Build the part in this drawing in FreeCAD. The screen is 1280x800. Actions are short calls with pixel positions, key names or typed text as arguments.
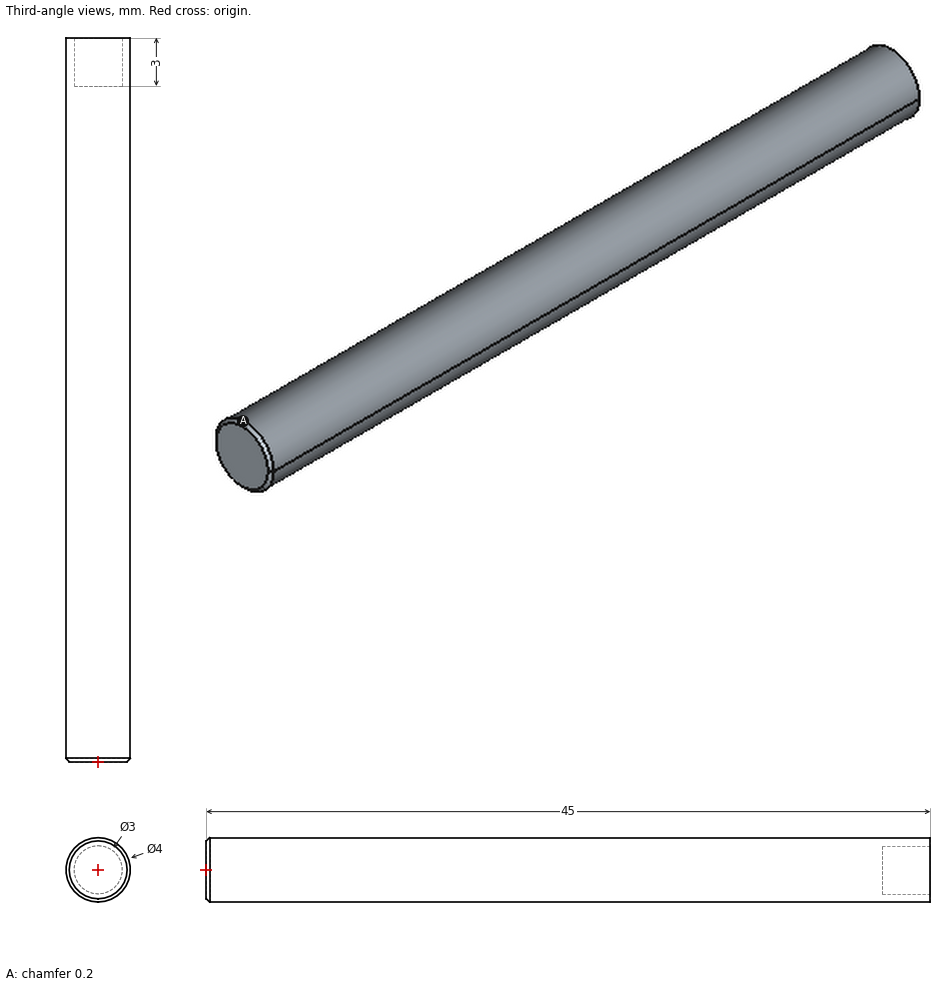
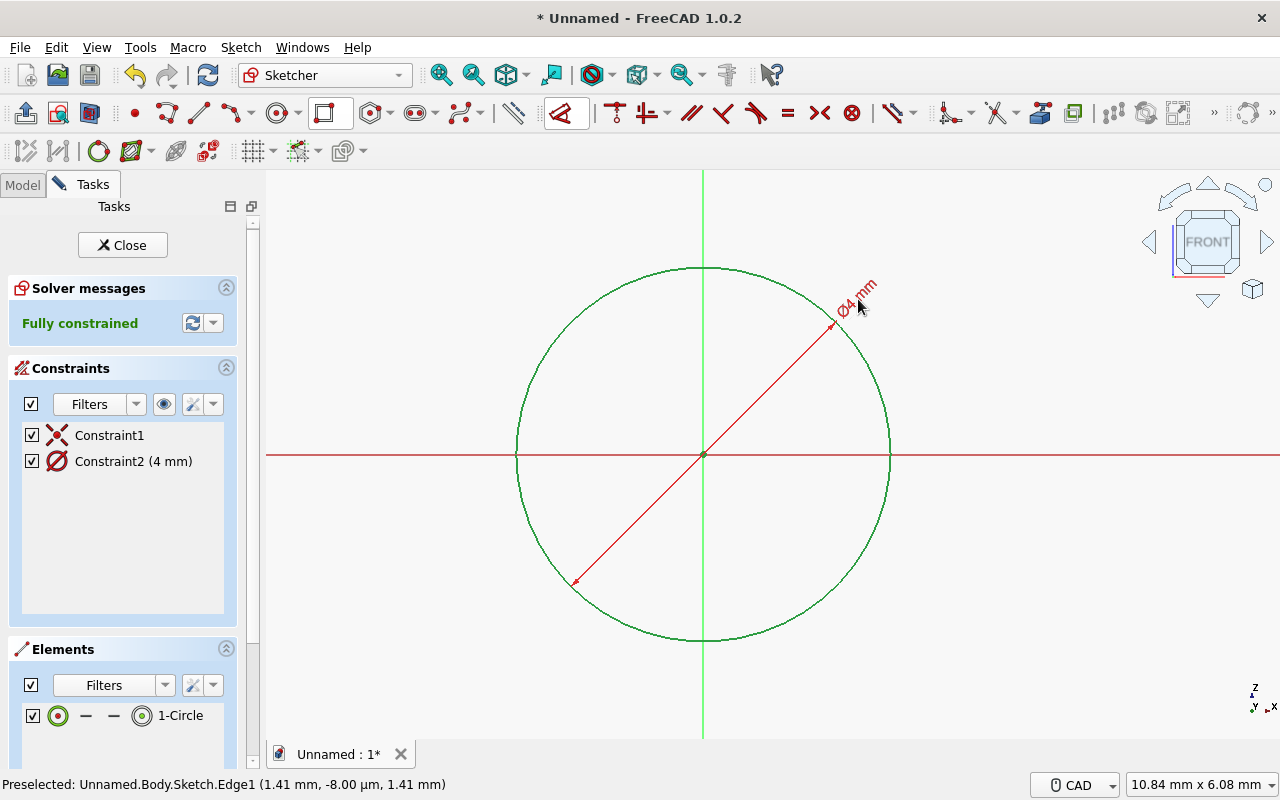
click(123, 245)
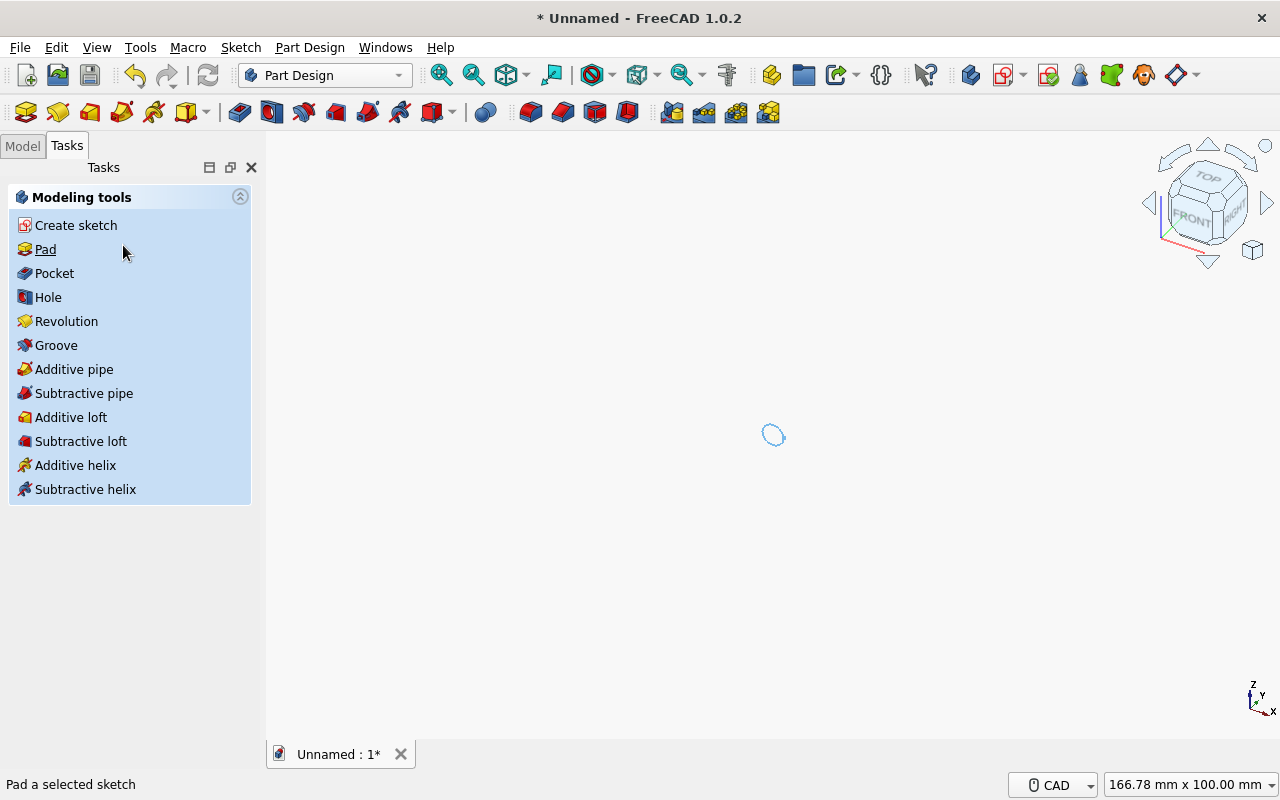
click(26, 112)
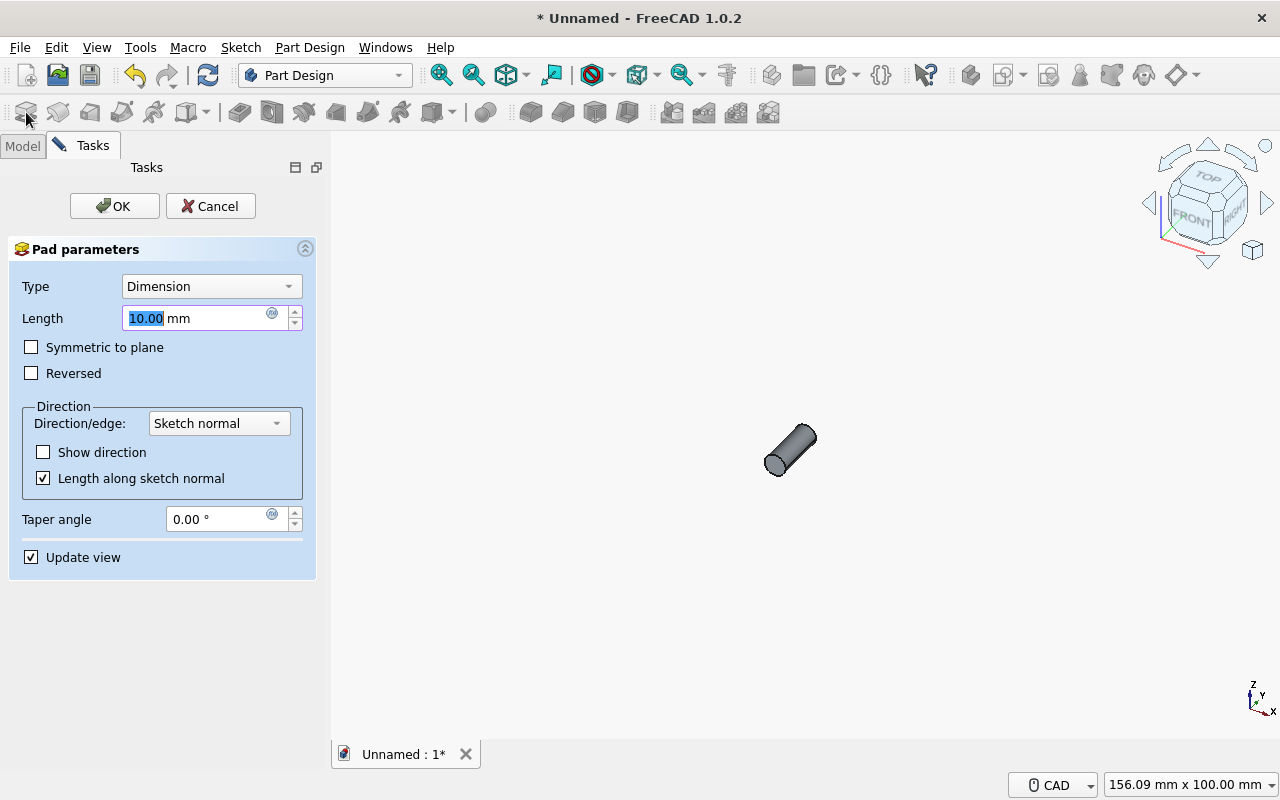
text(45)
key(Tab)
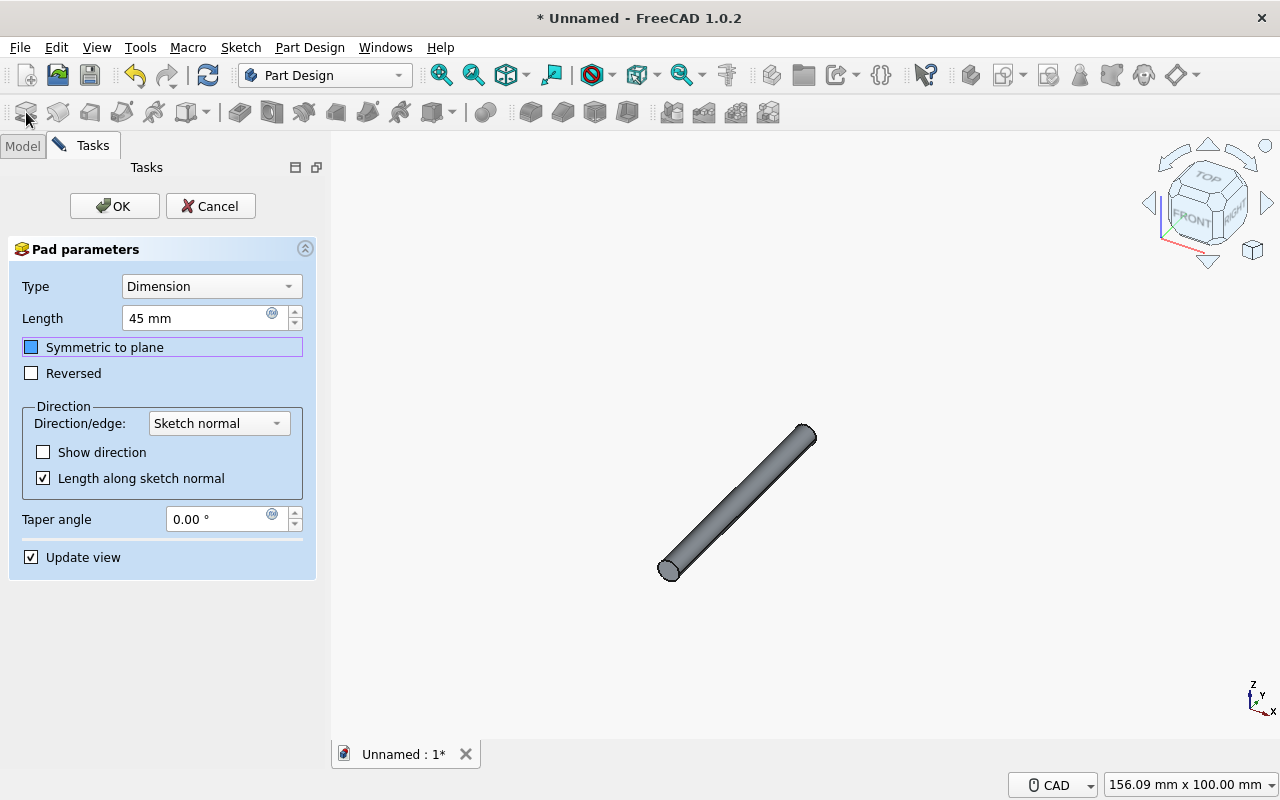
click(30, 373)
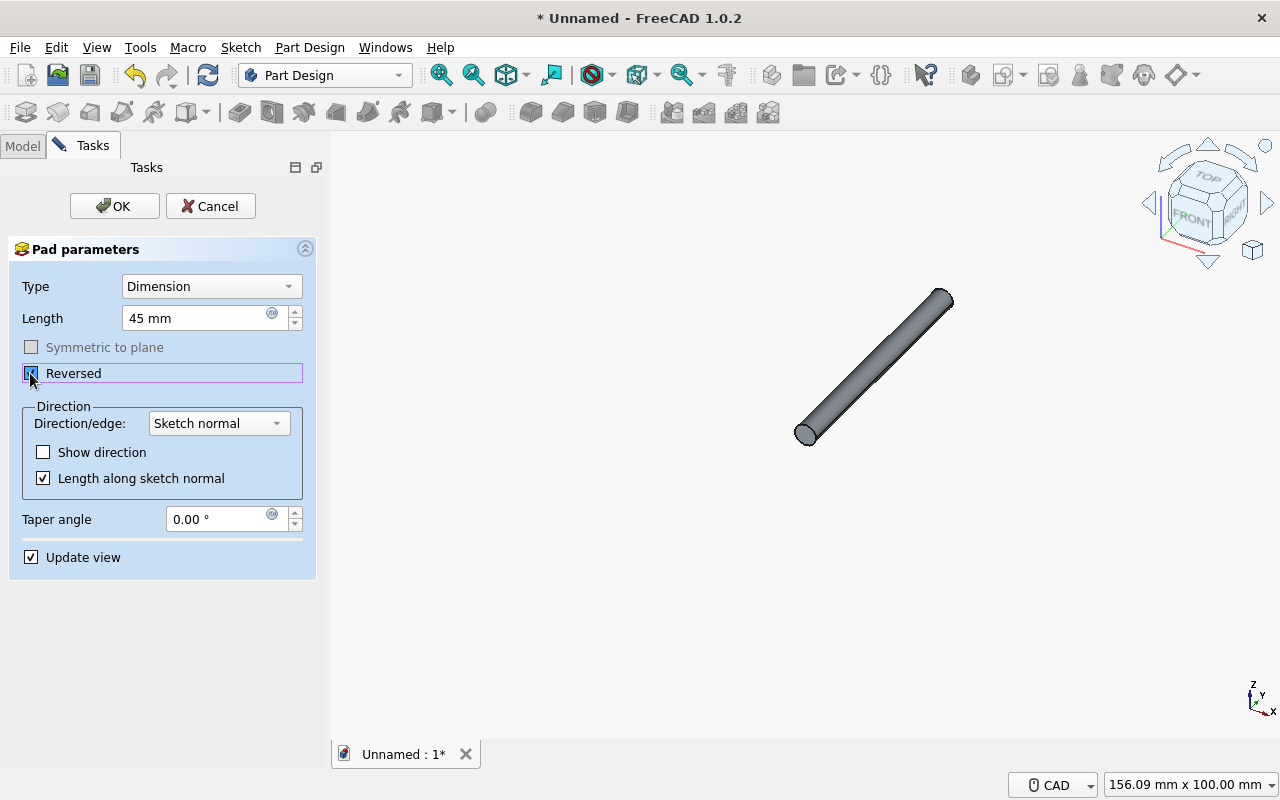
click(115, 206)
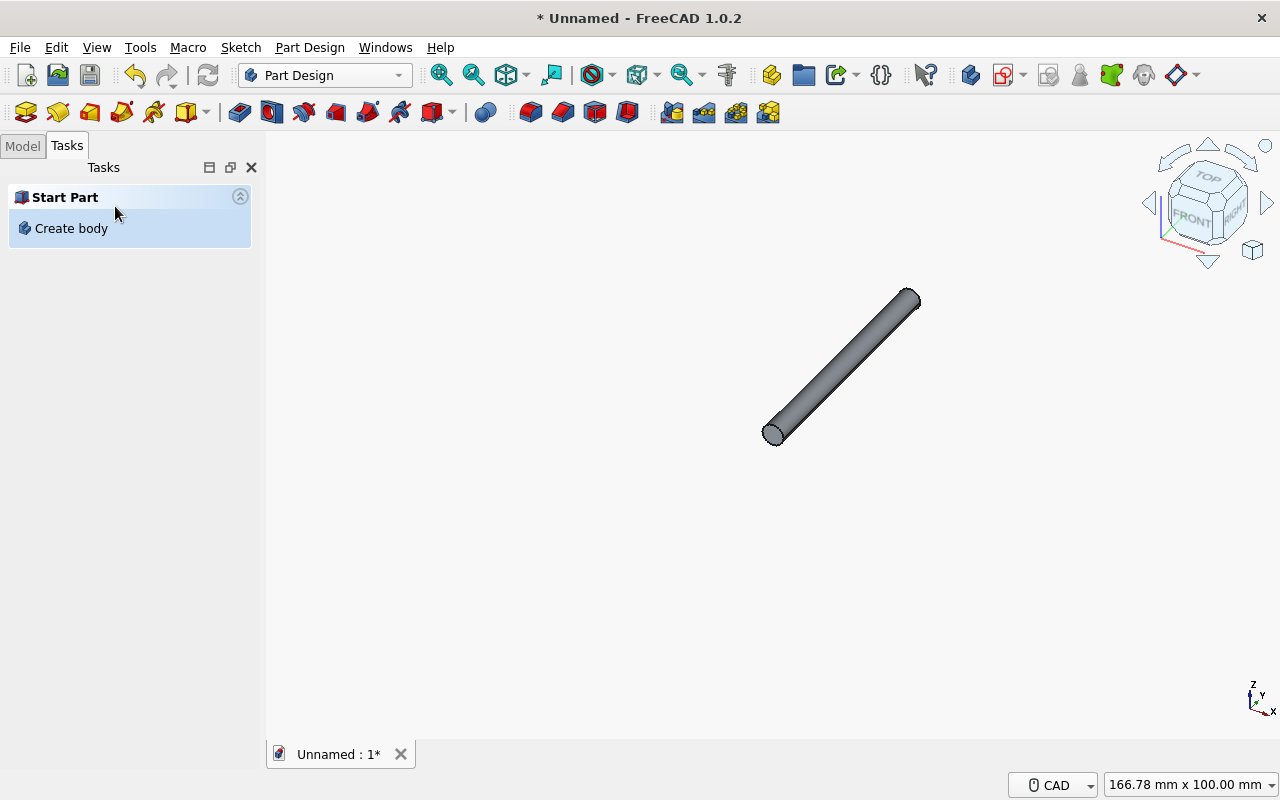
key(v)
key(f)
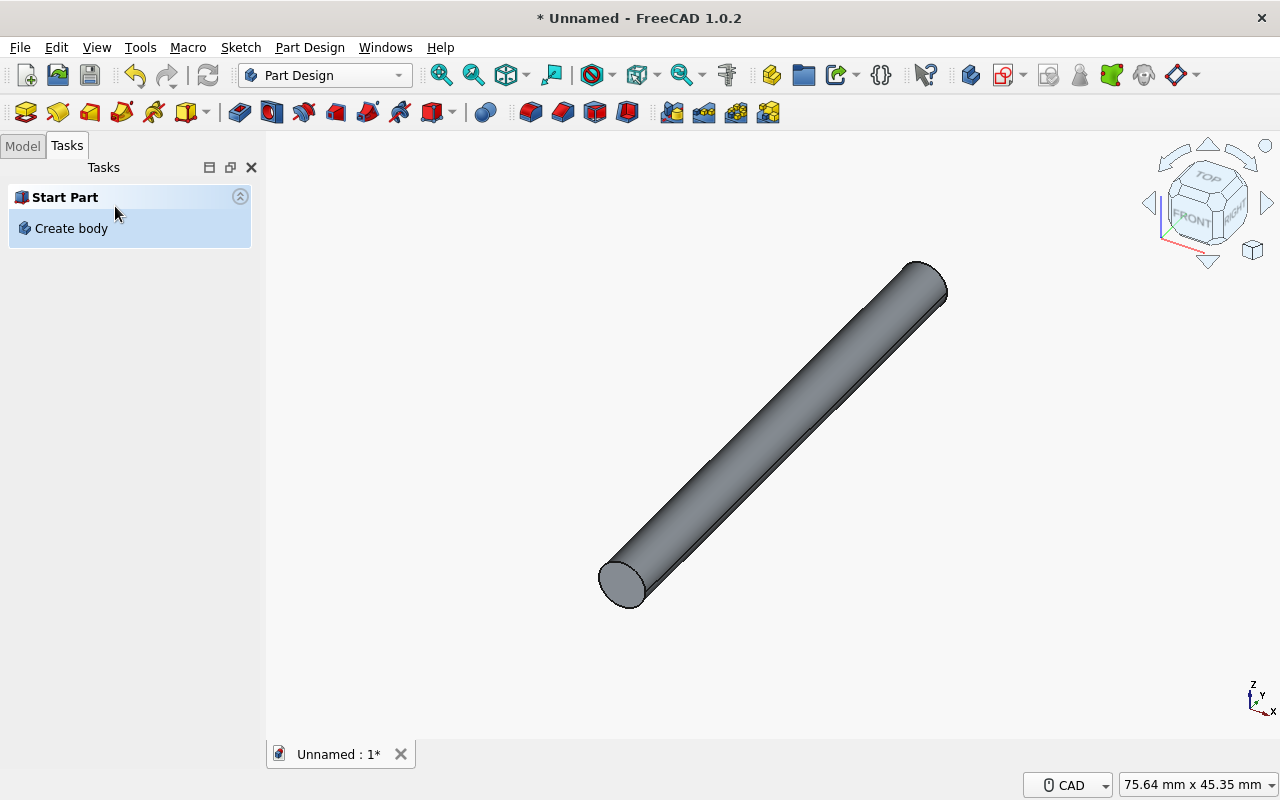
click(603, 565)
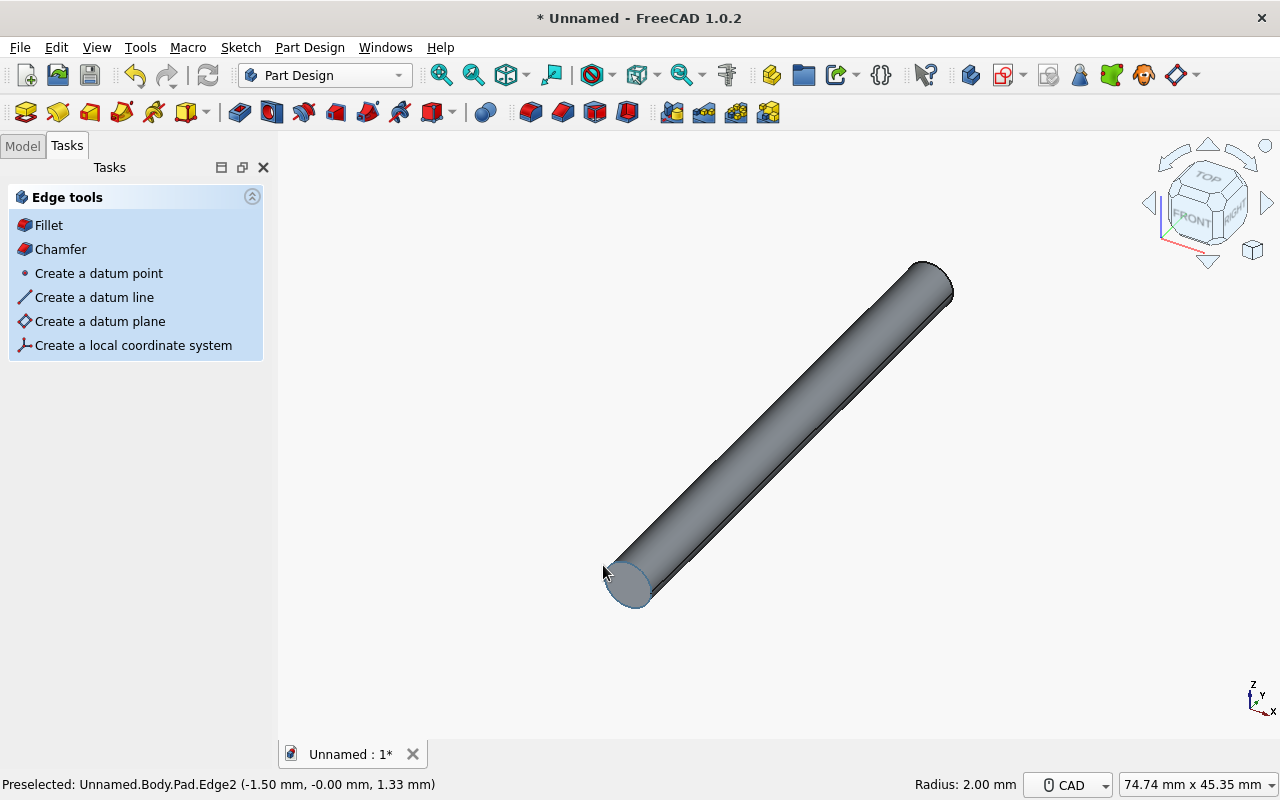
click(564, 112)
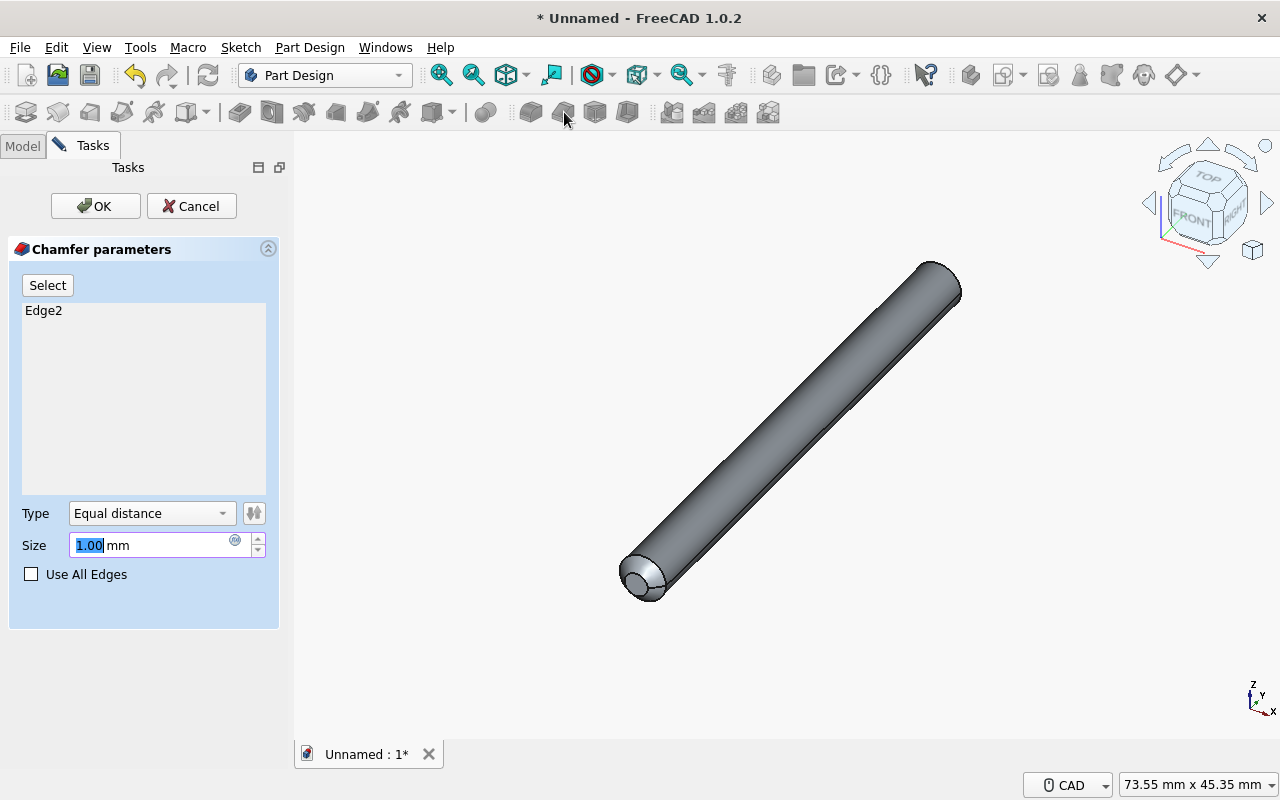
text(0.2)
key(Tab)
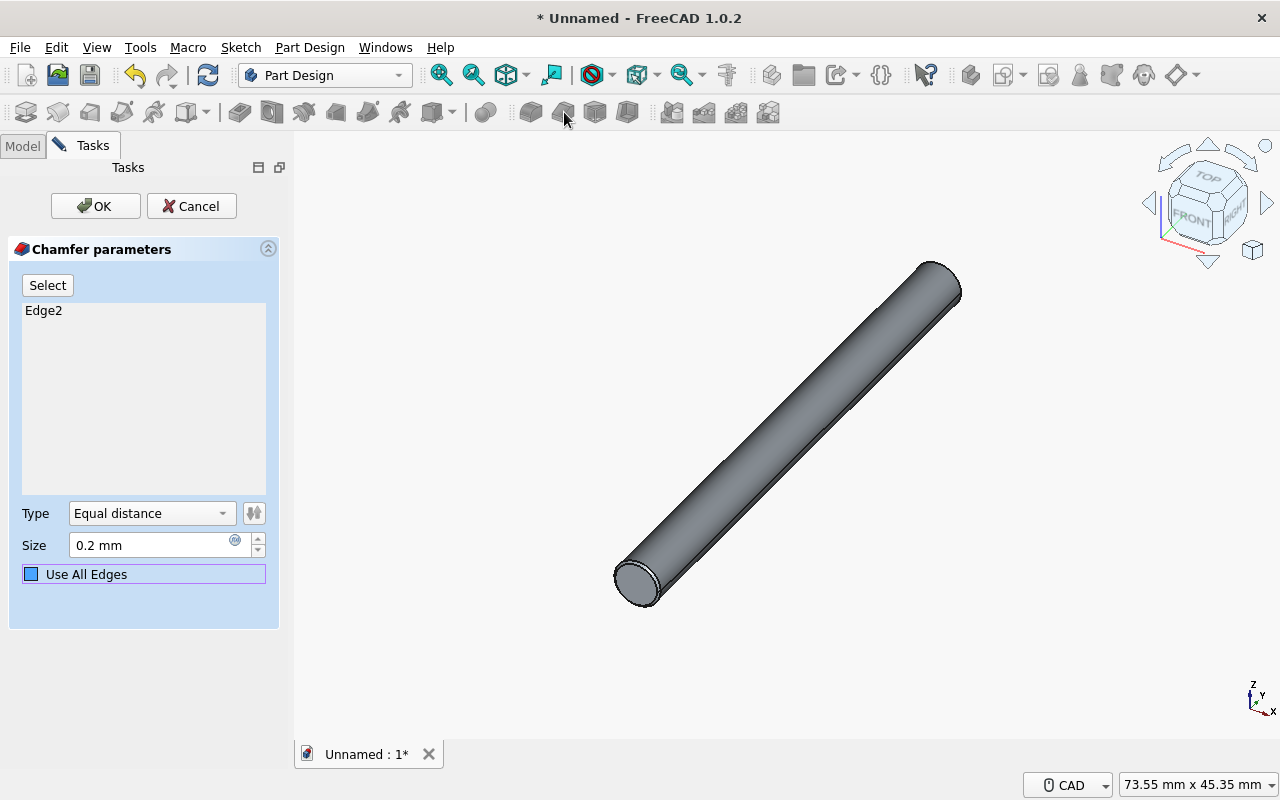
click(96, 206)